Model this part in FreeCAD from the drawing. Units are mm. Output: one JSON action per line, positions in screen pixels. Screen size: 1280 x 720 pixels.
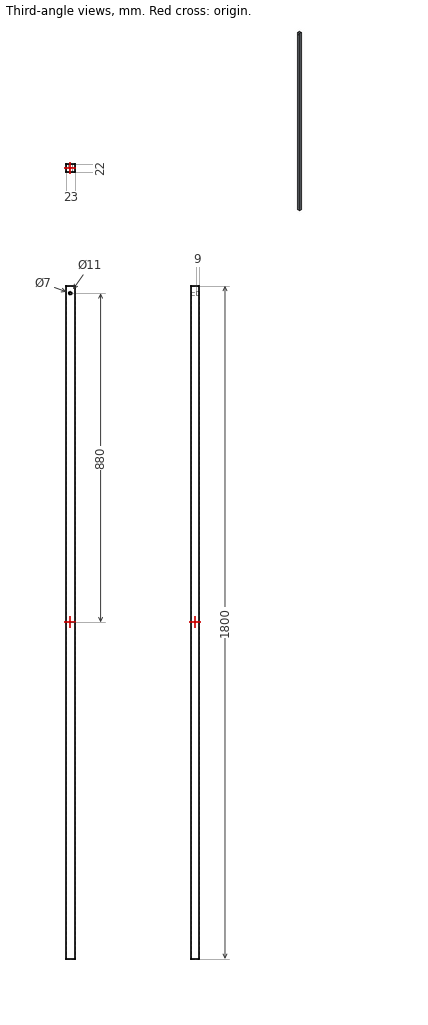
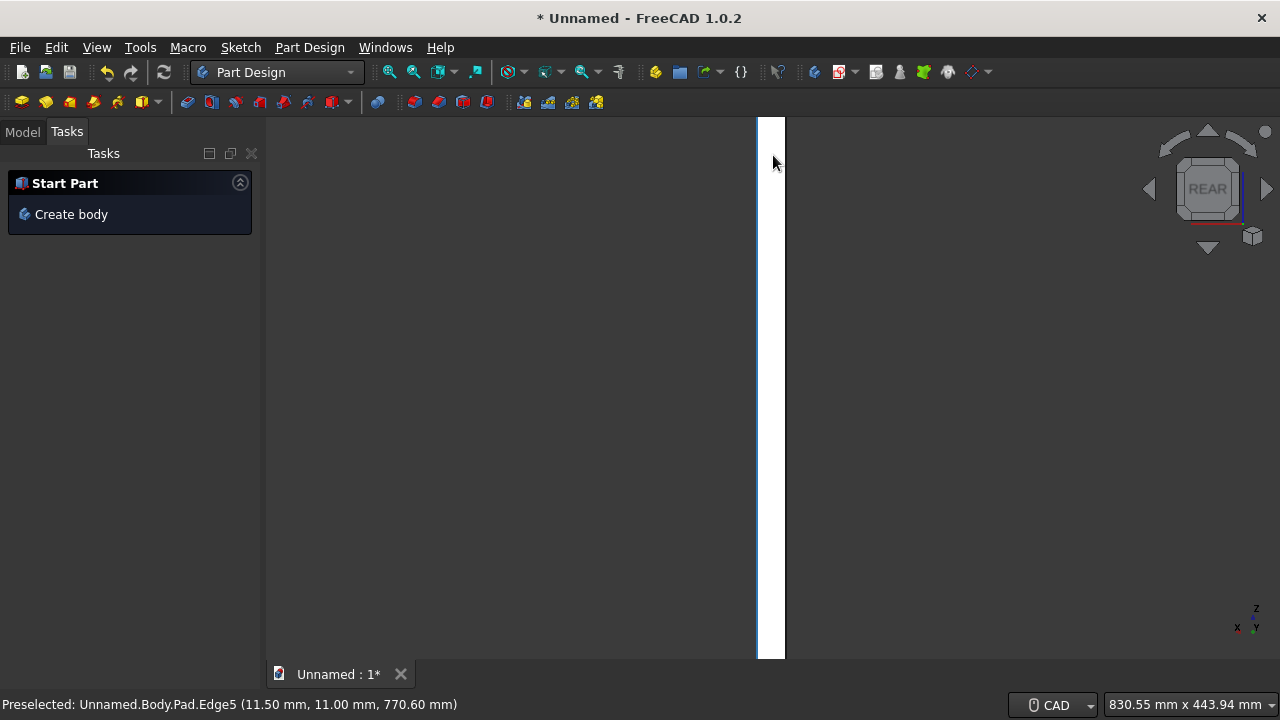
{"action": "left_click", "coordinate": [771, 157]}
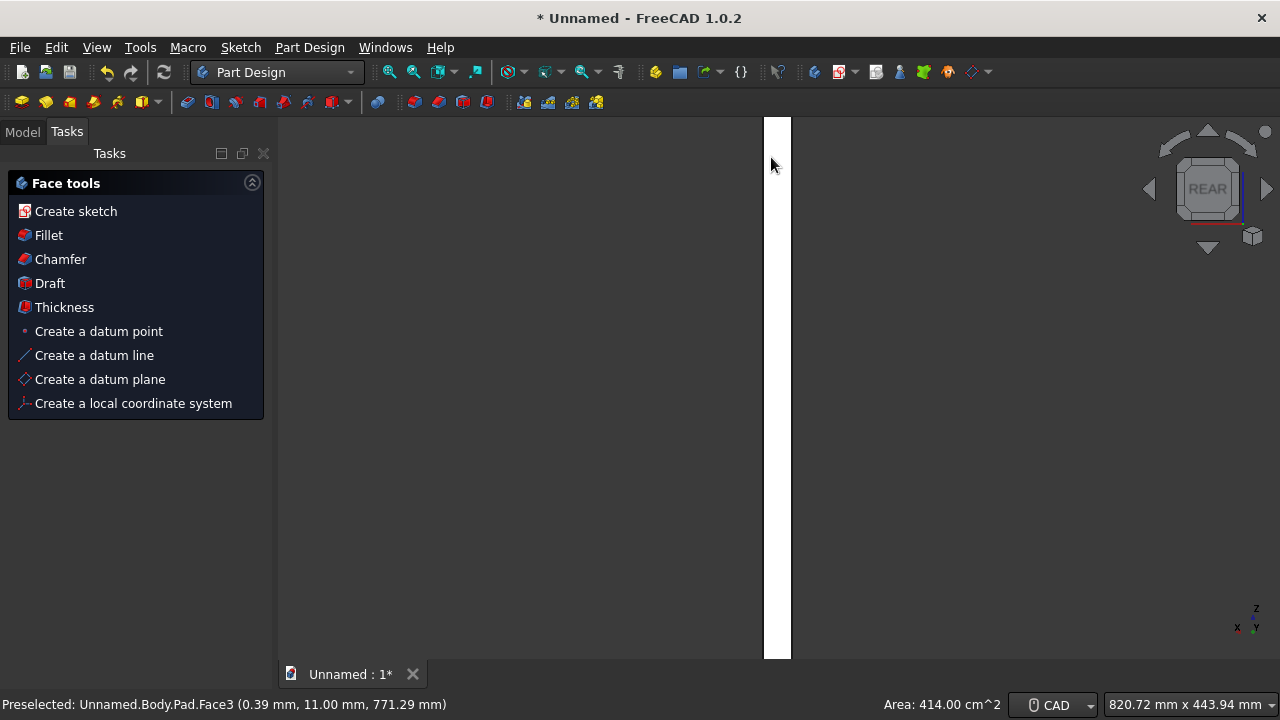
{"action": "left_click", "coordinate": [840, 72]}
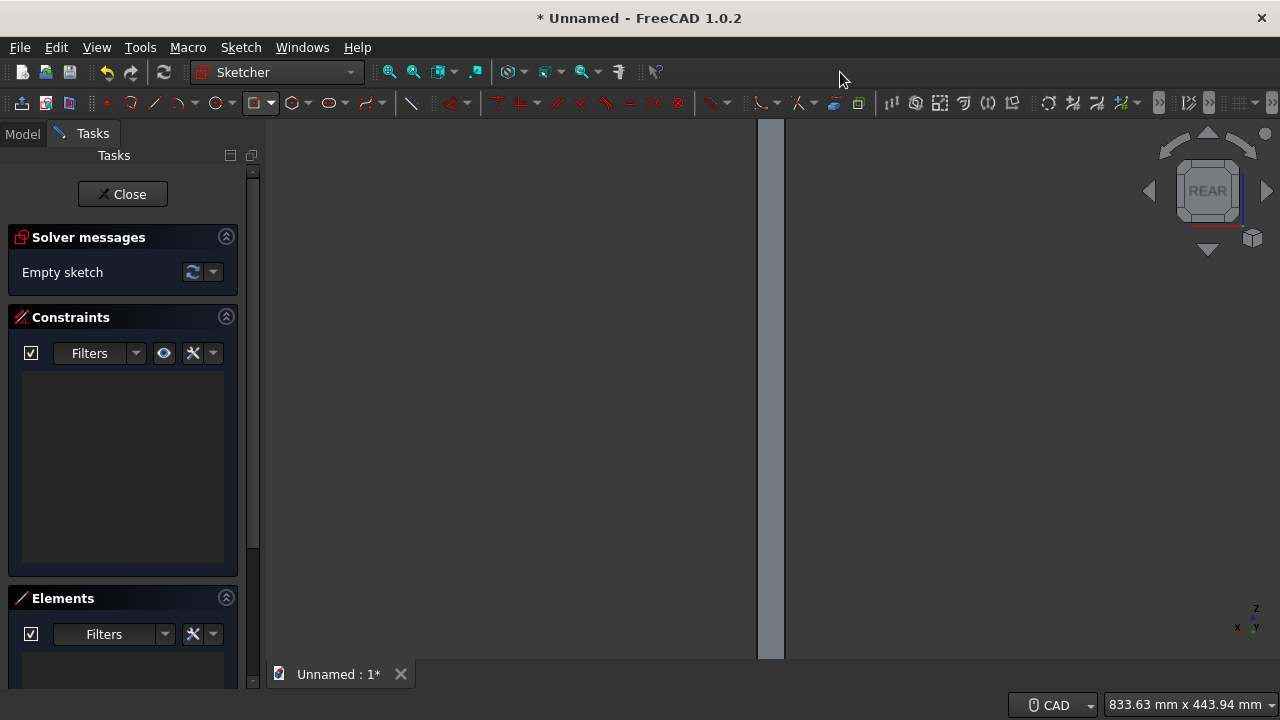
{"action": "scroll", "coordinate": [704, 389], "scroll_direction": "down", "scroll_amount": 5}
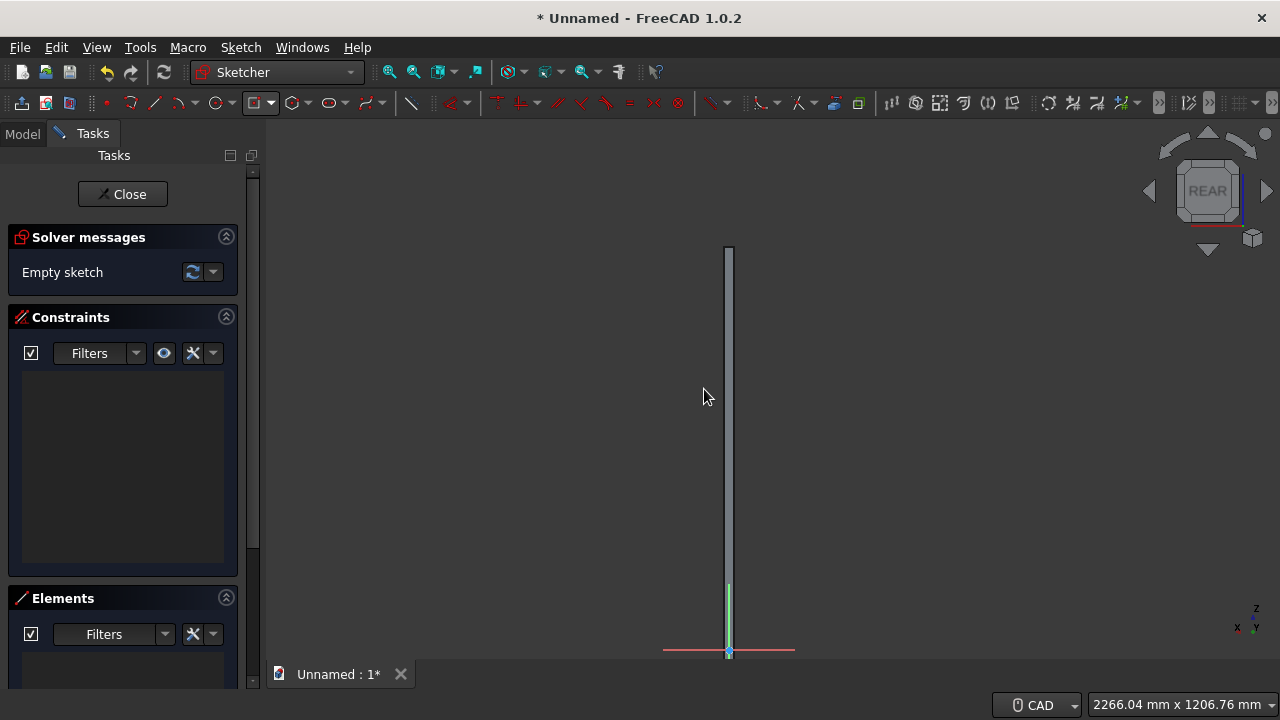
{"action": "scroll", "coordinate": [730, 249], "scroll_direction": "up", "scroll_amount": 15}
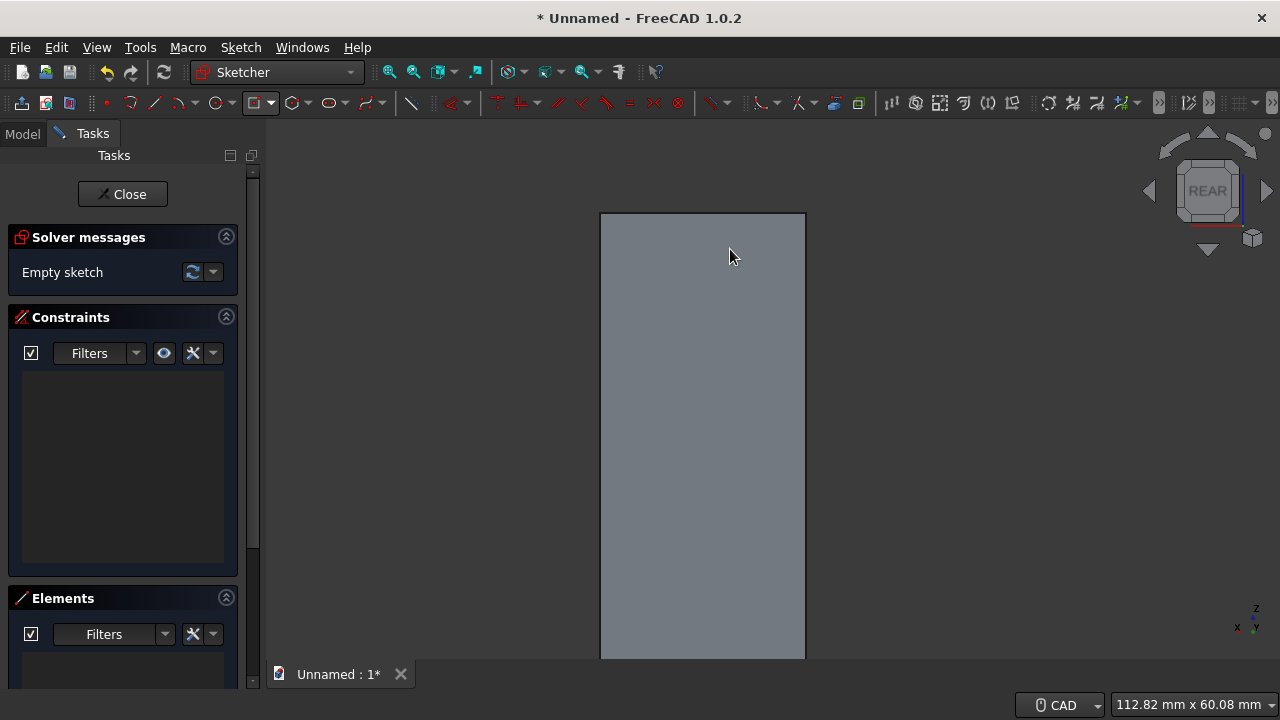
{"action": "scroll", "coordinate": [703, 394], "scroll_direction": "up", "scroll_amount": 6}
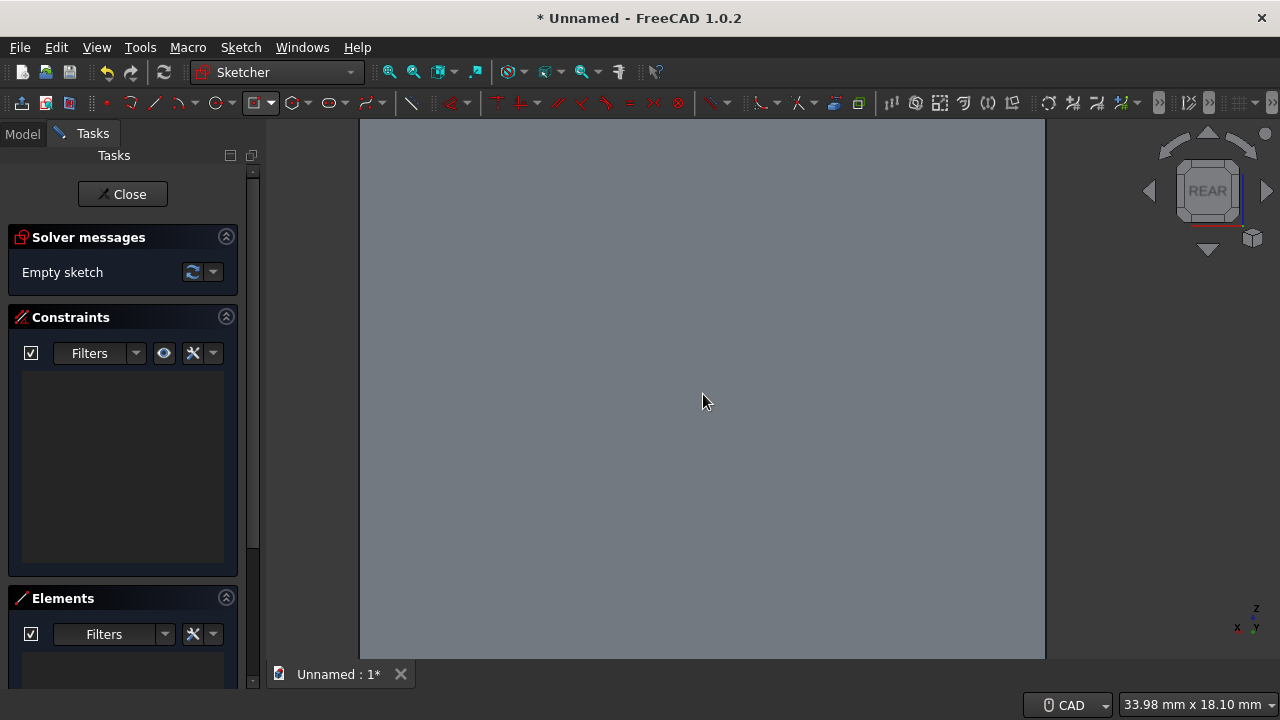
{"action": "left_click", "coordinate": [216, 104]}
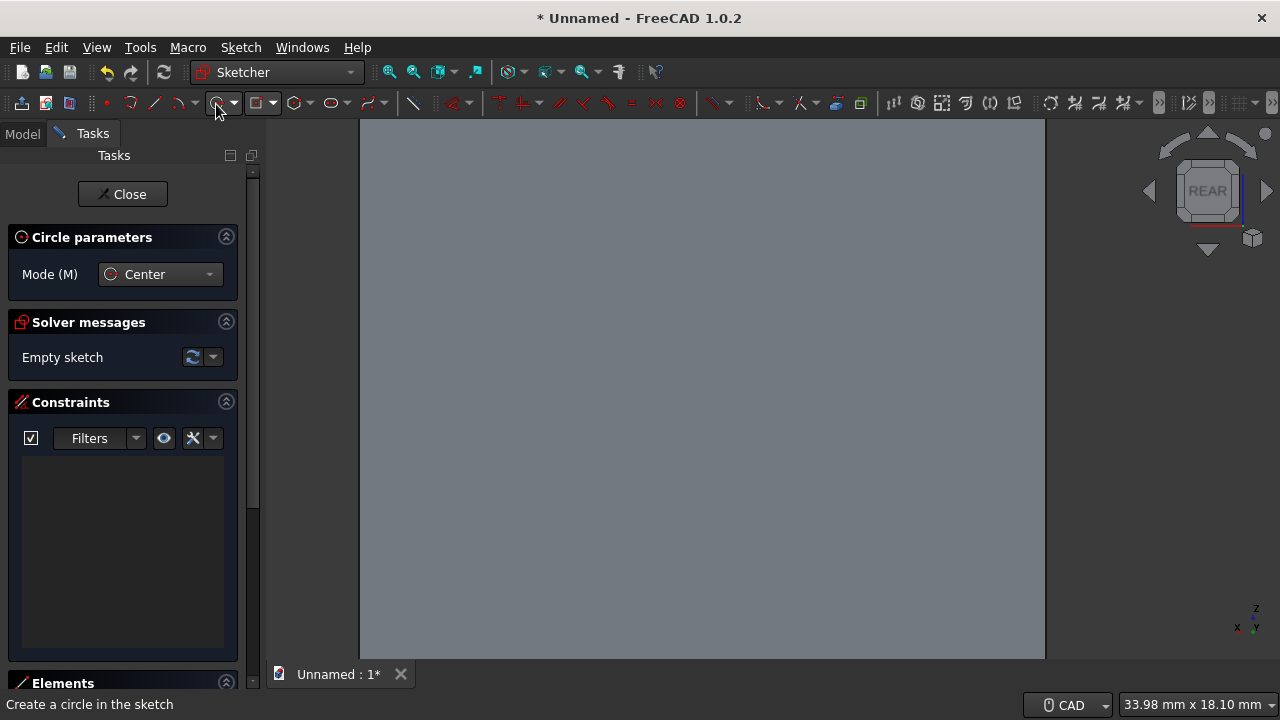
{"action": "left_click", "coordinate": [702, 388]}
{"action": "left_click", "coordinate": [818, 272]}
{"action": "key", "text": "Escape"}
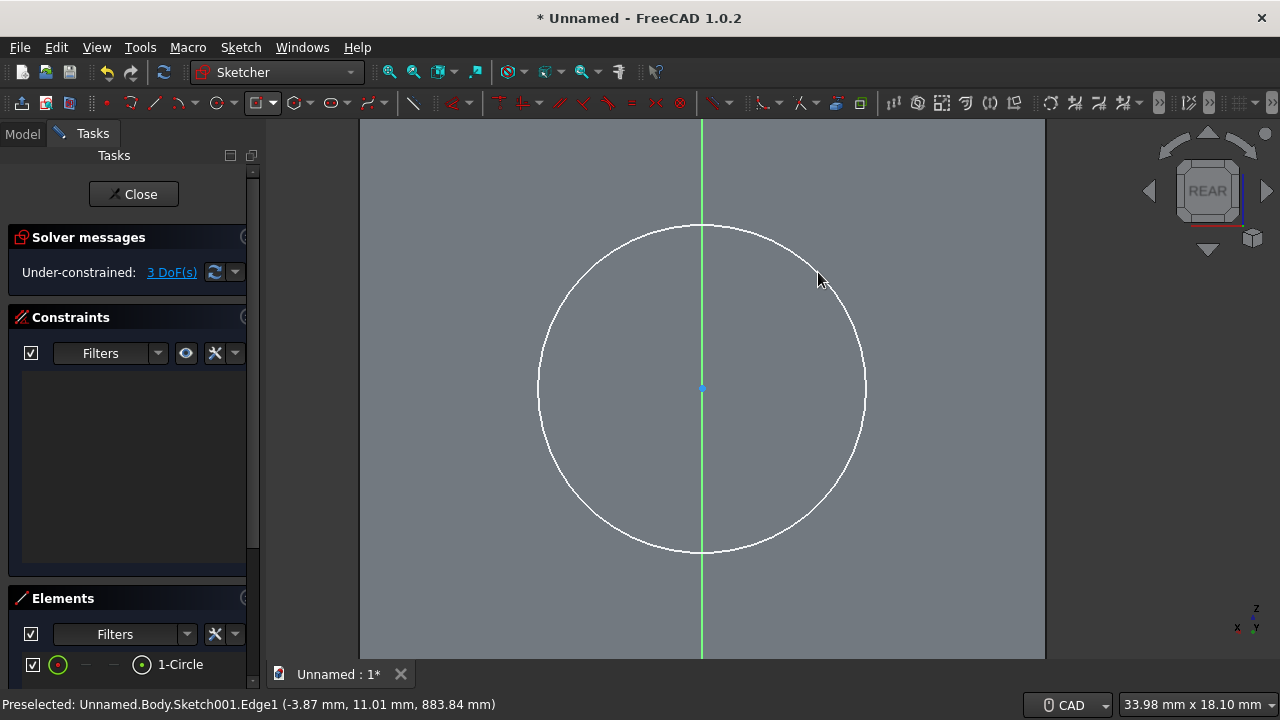
{"action": "left_click", "coordinate": [702, 389]}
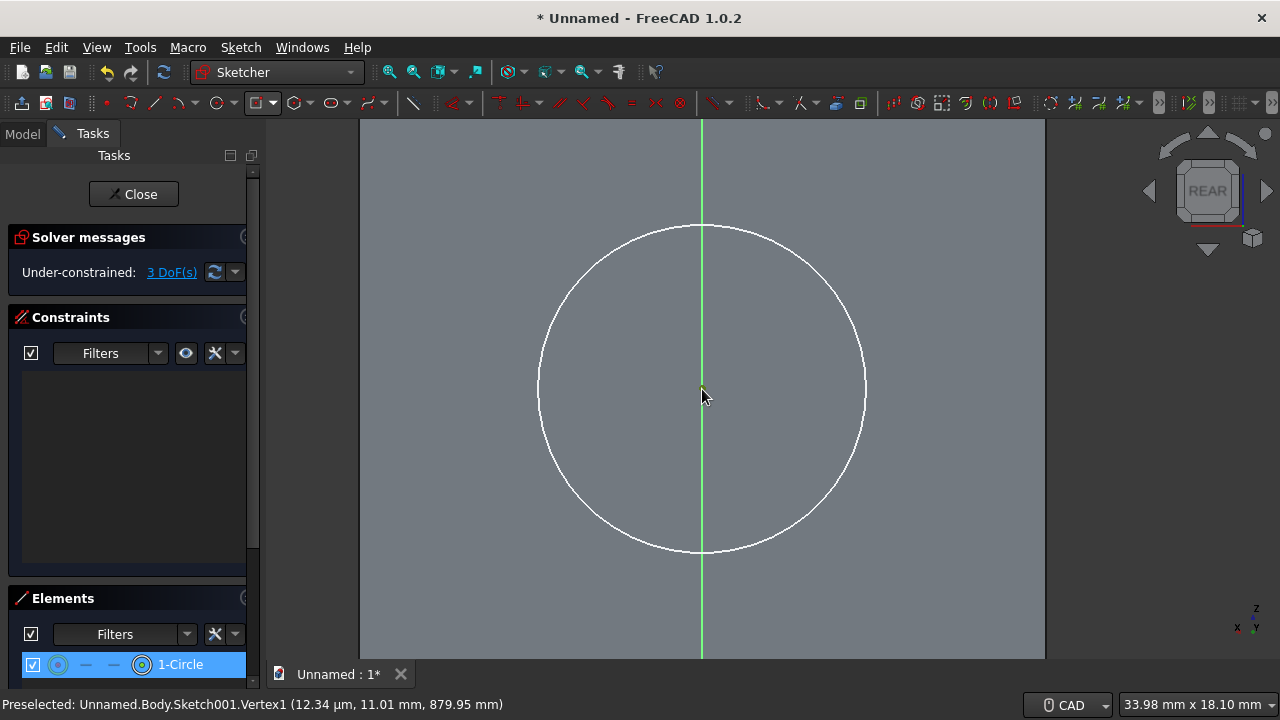
{"action": "left_click", "coordinate": [702, 596]}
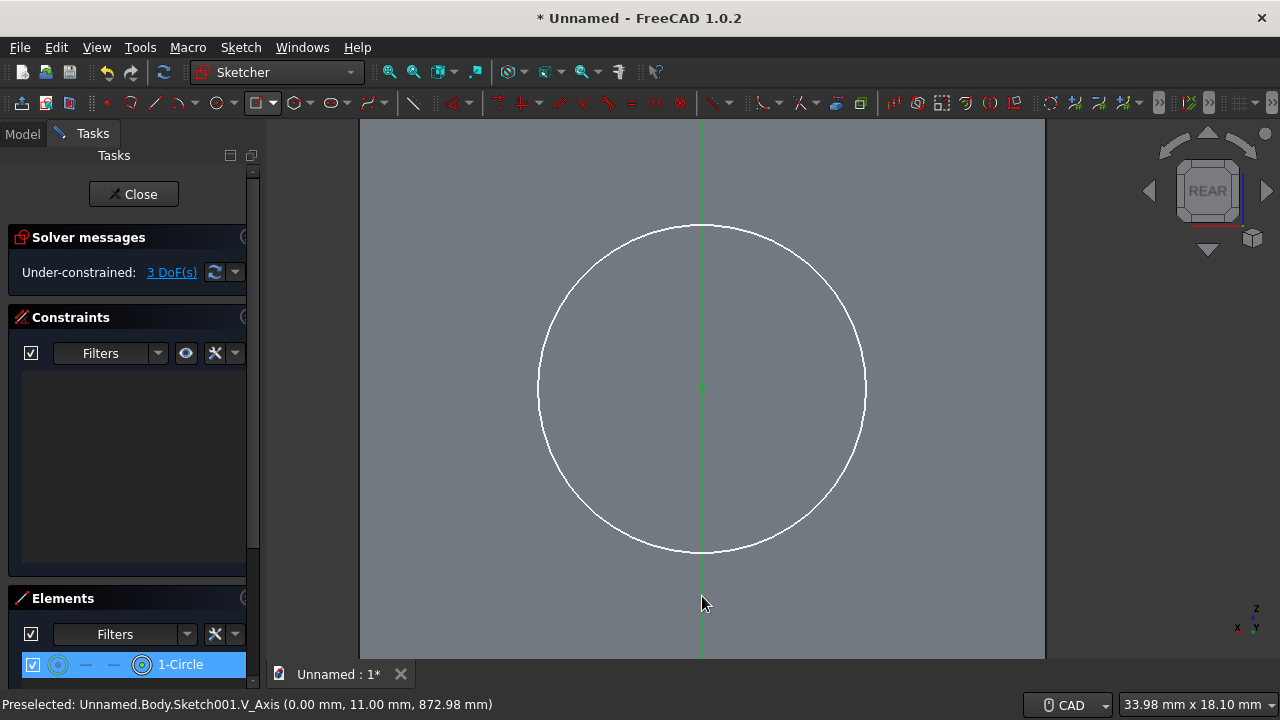
{"action": "left_click", "coordinate": [500, 104]}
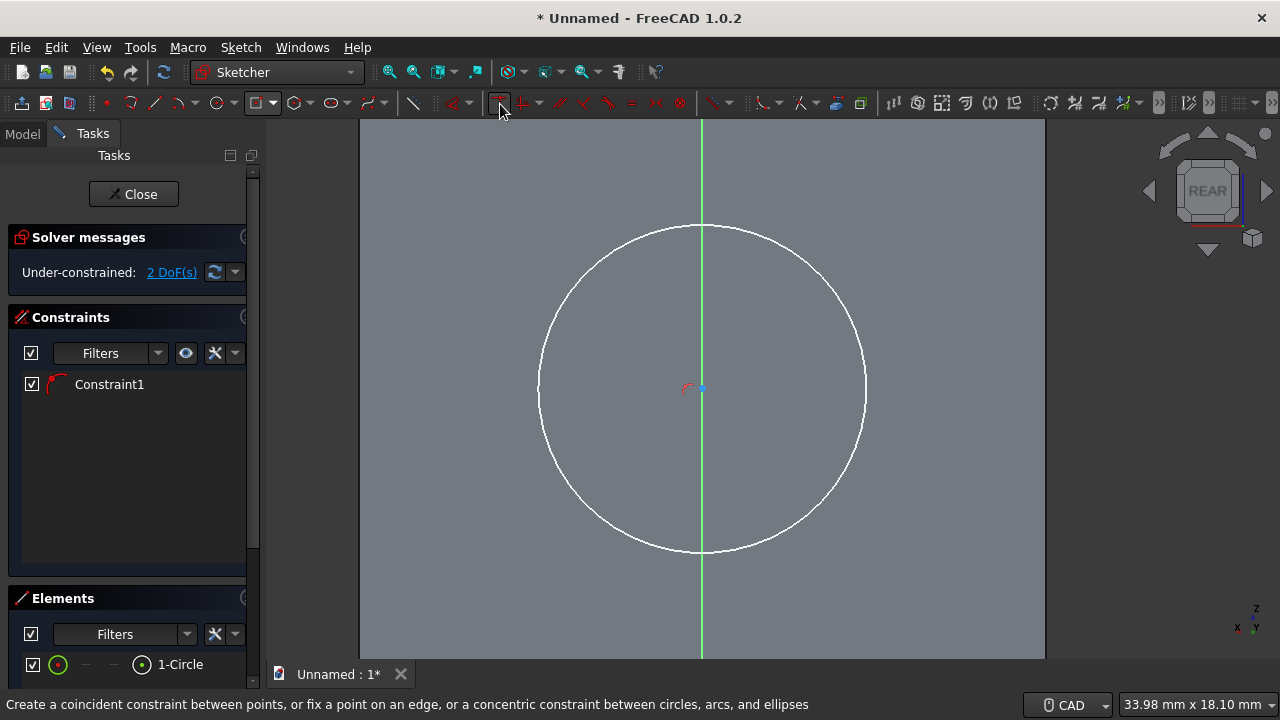
{"action": "left_click", "coordinate": [452, 104]}